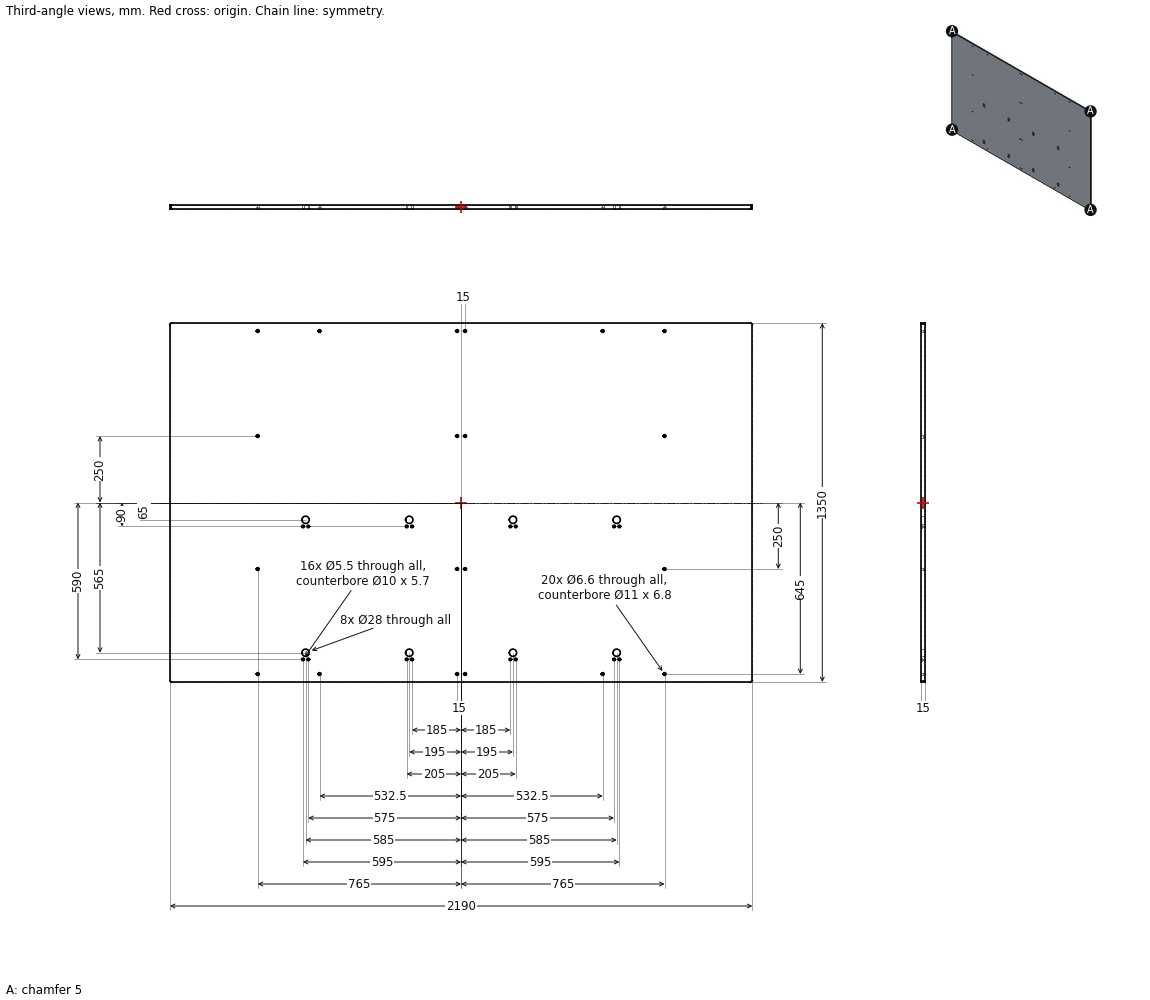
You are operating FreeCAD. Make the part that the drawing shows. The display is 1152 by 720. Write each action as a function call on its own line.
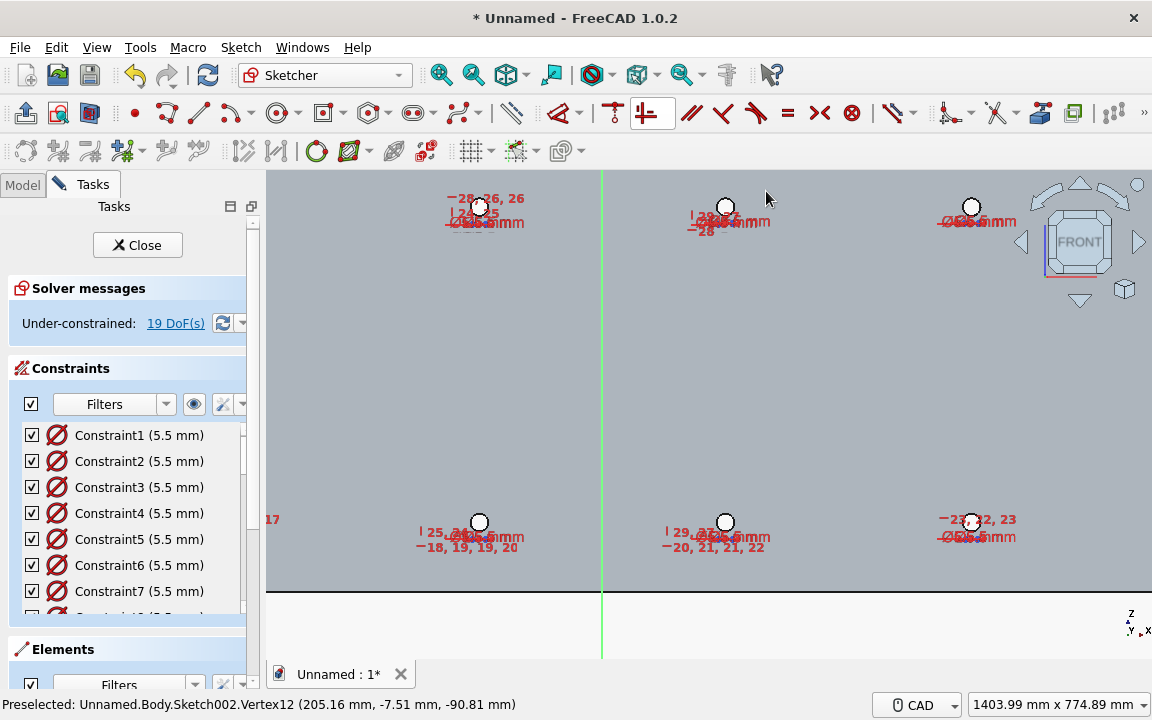
scroll(719, 225, up, 4)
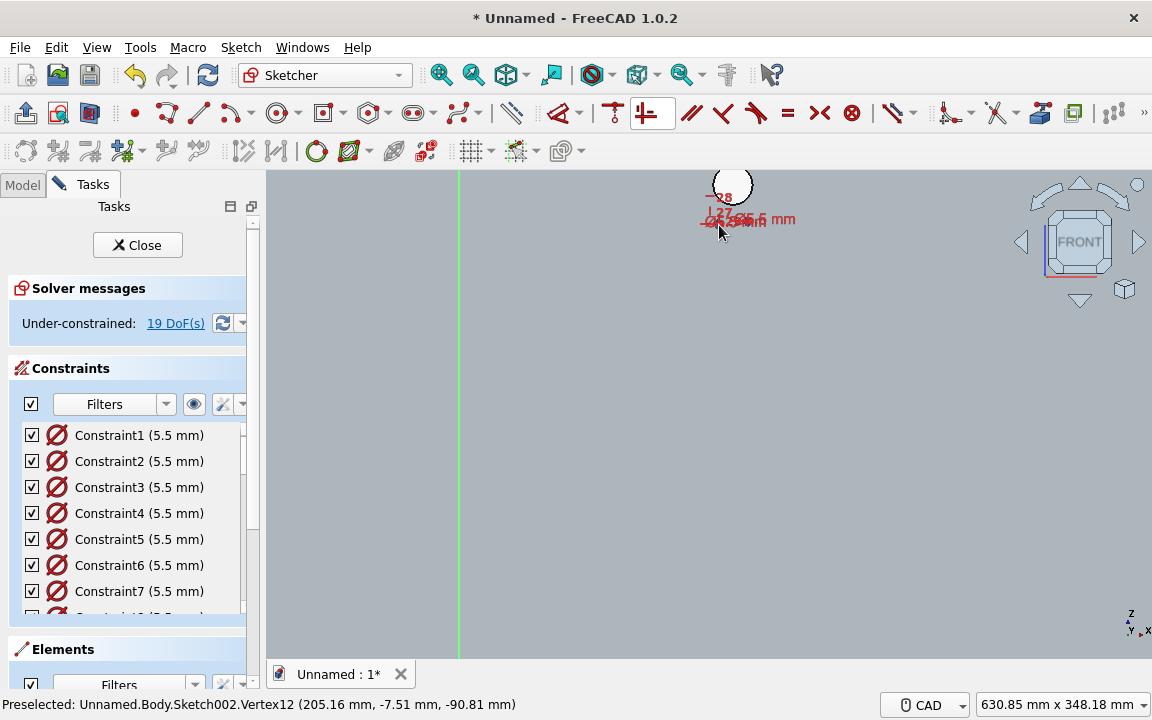
scroll(718, 224, up, 4)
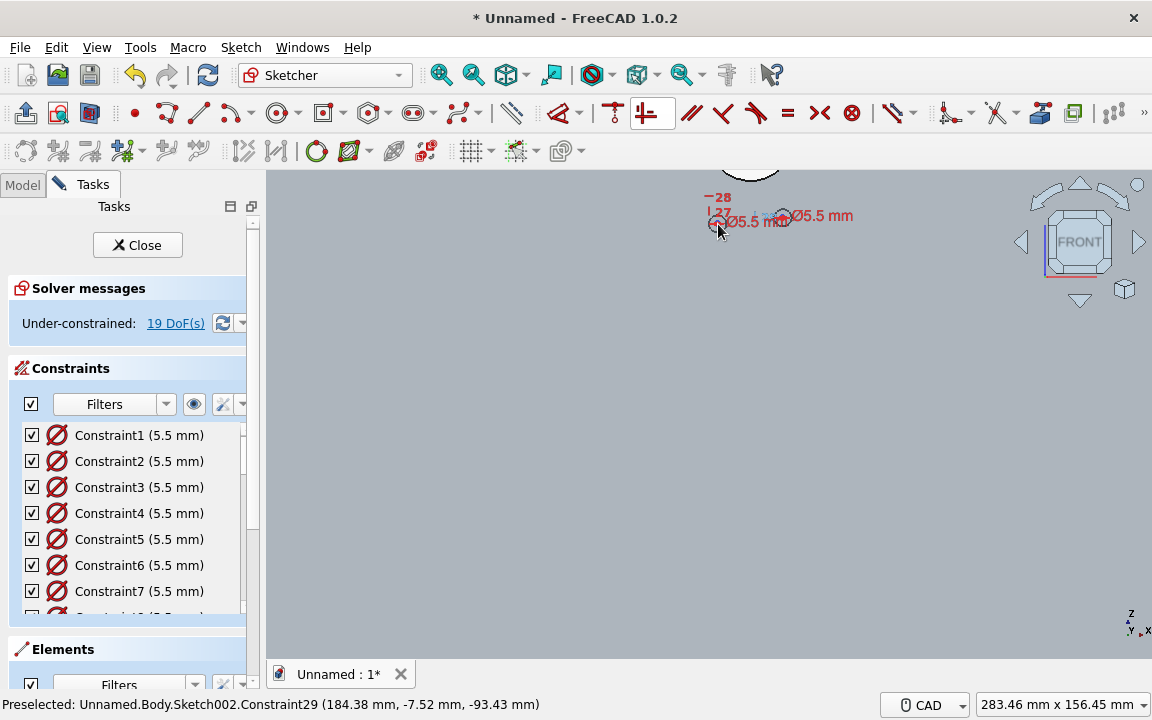
click(718, 224)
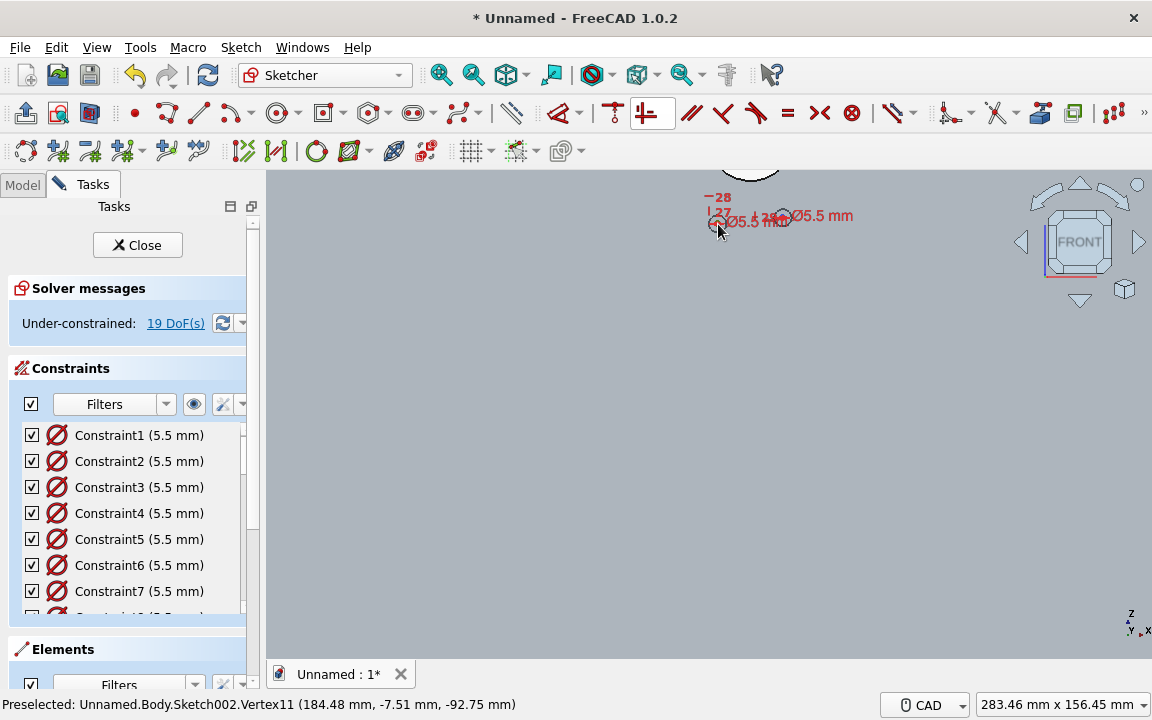
scroll(719, 345, down, 10)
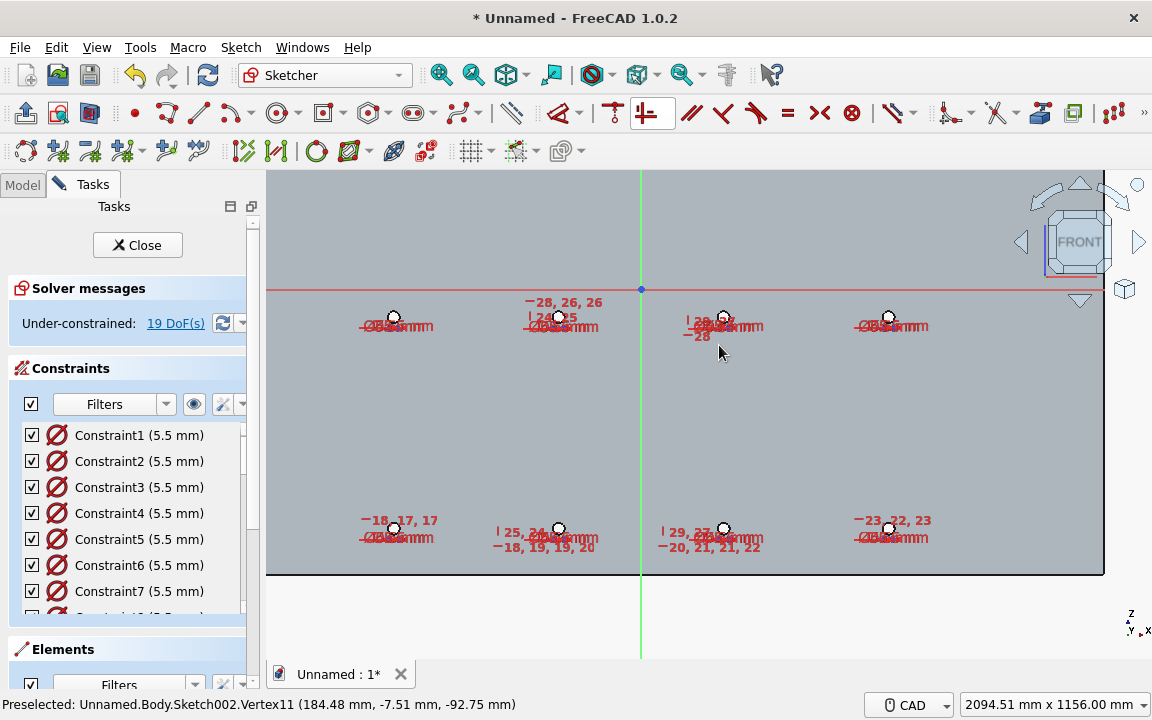
scroll(728, 328, up, 2)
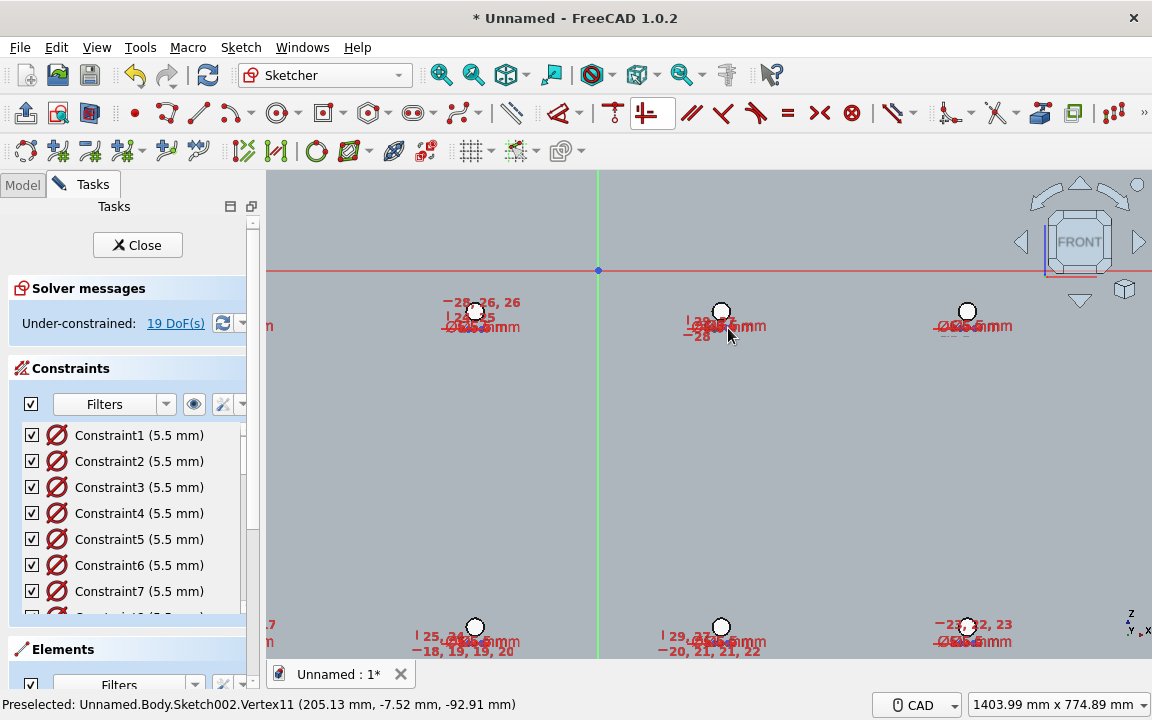
scroll(728, 328, up, 4)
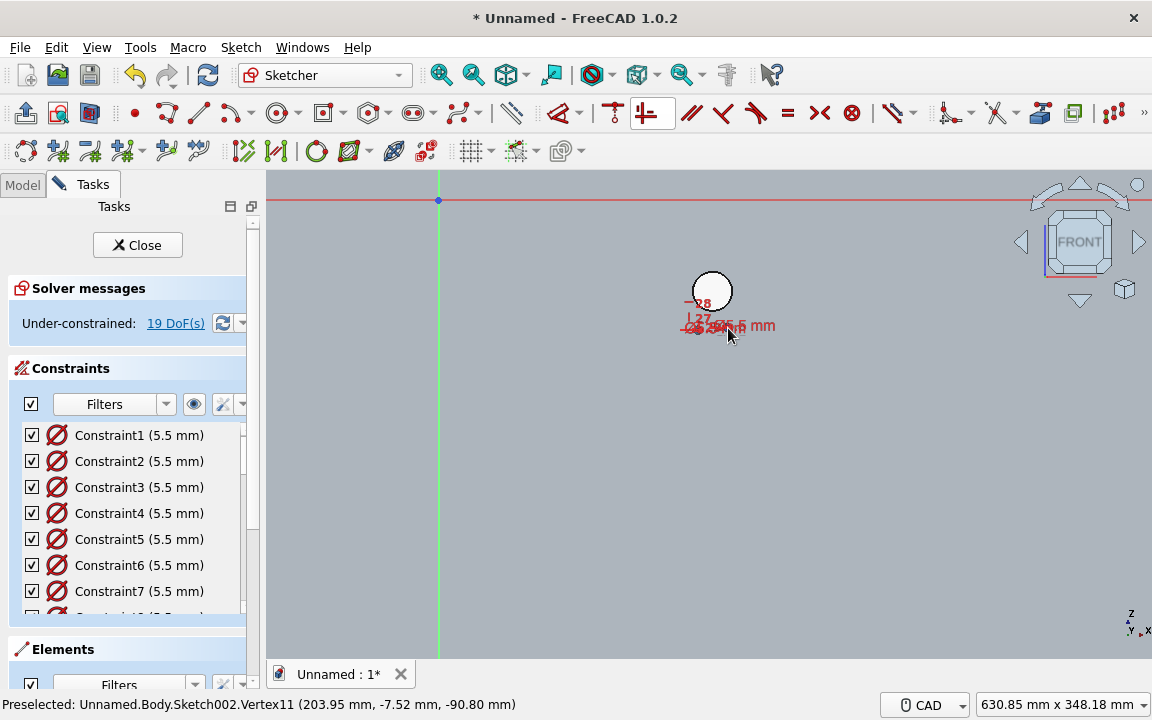
click(727, 328)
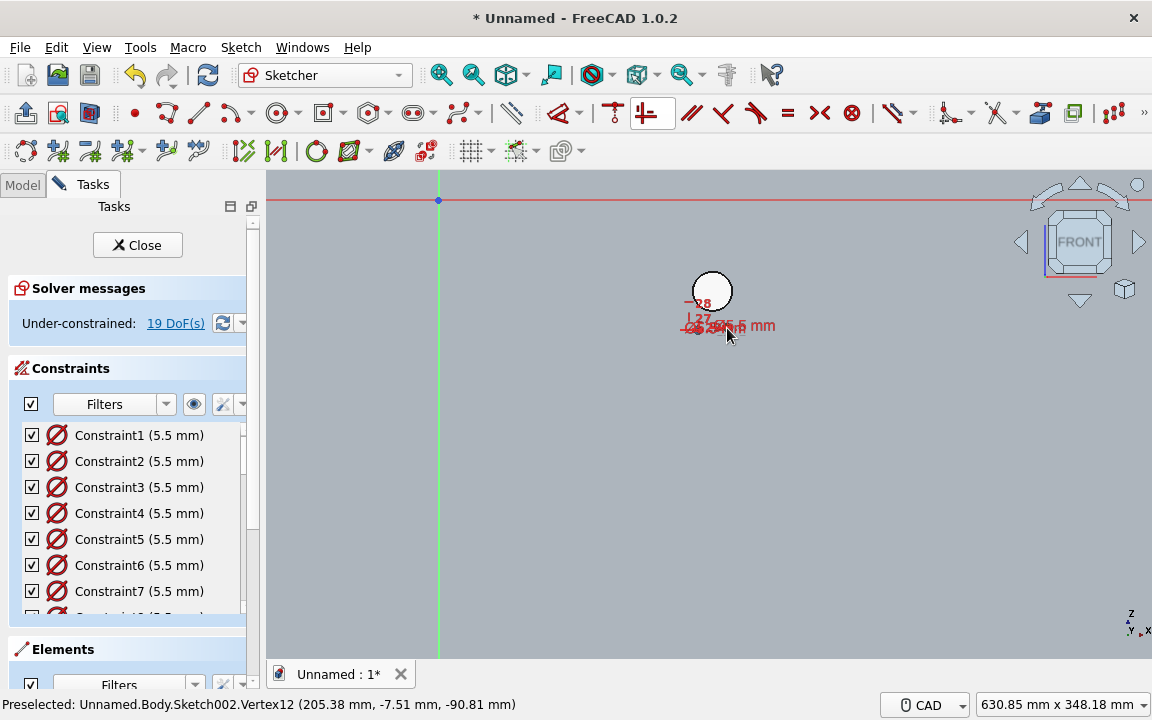
key(h)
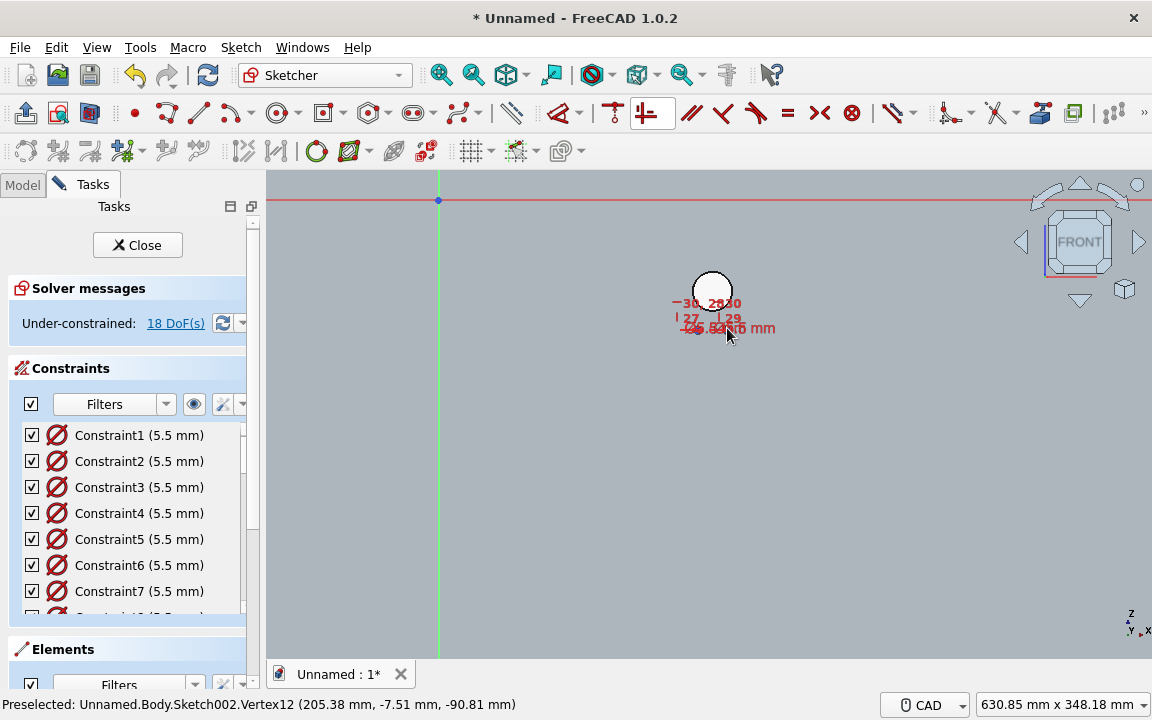
scroll(727, 328, down, 6)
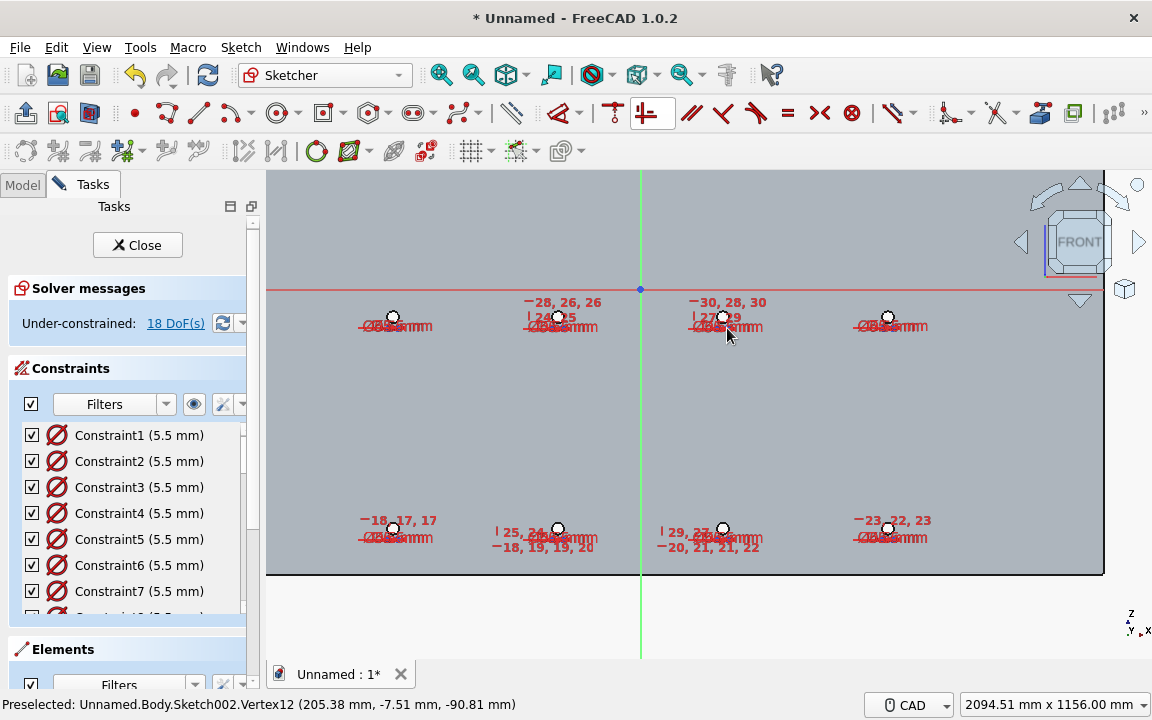
scroll(884, 540, up, 2)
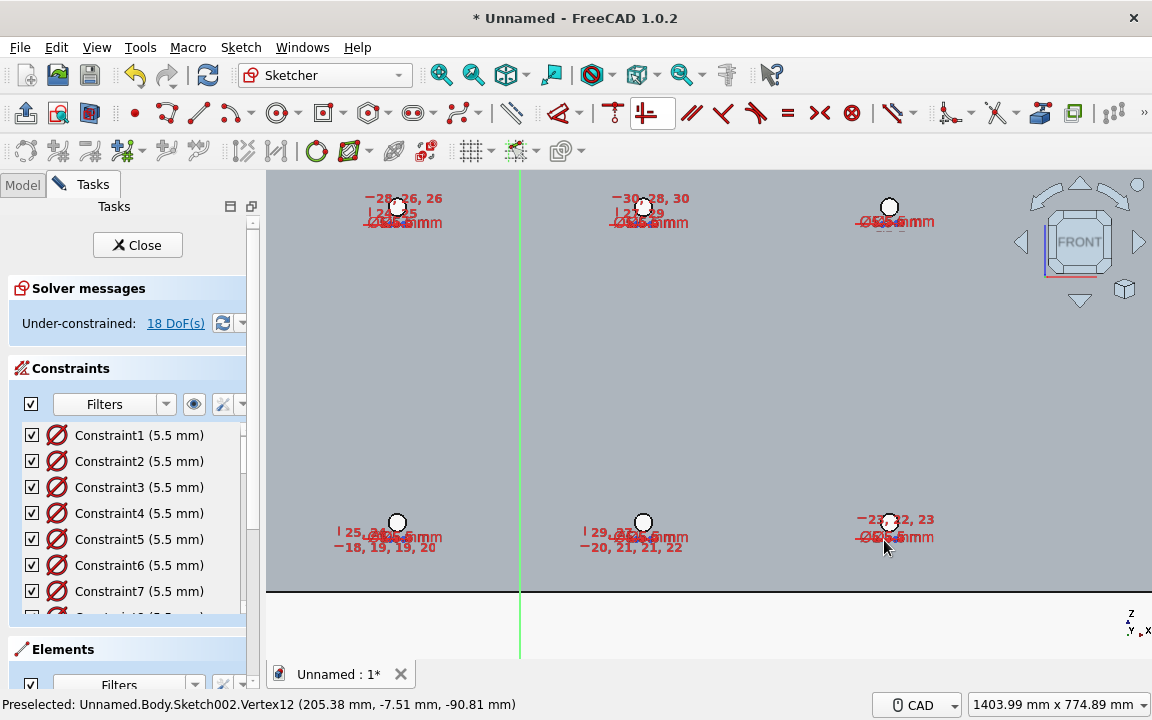
click(883, 539)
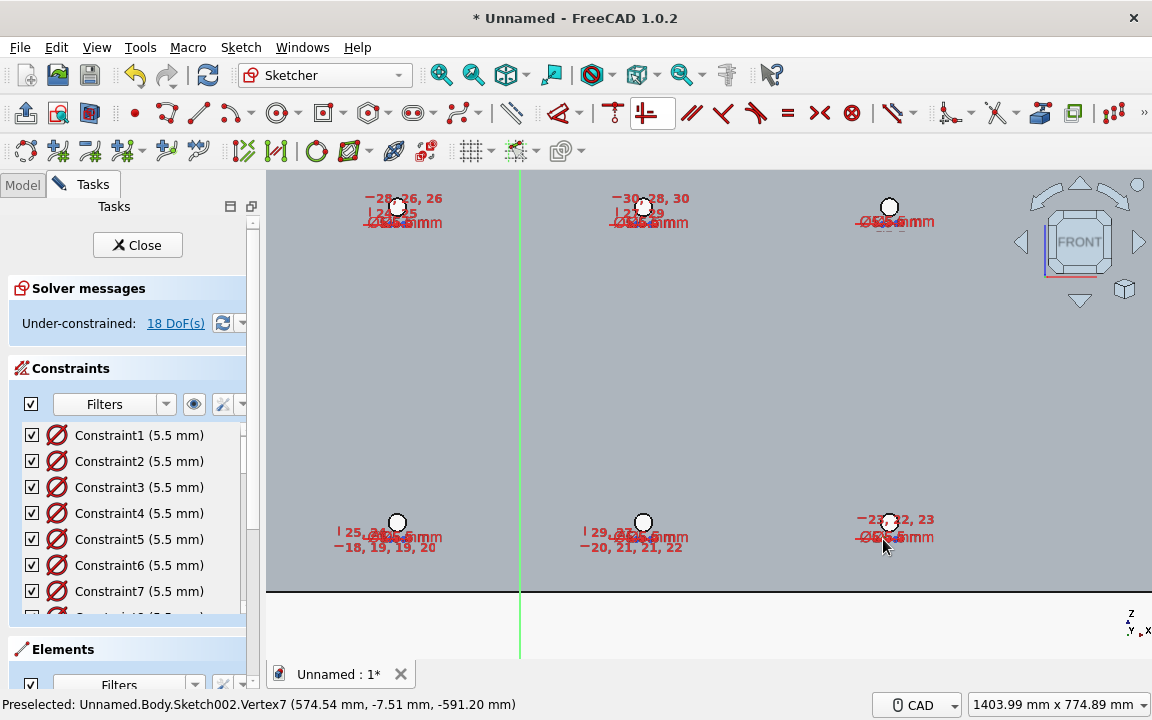
click(883, 224)